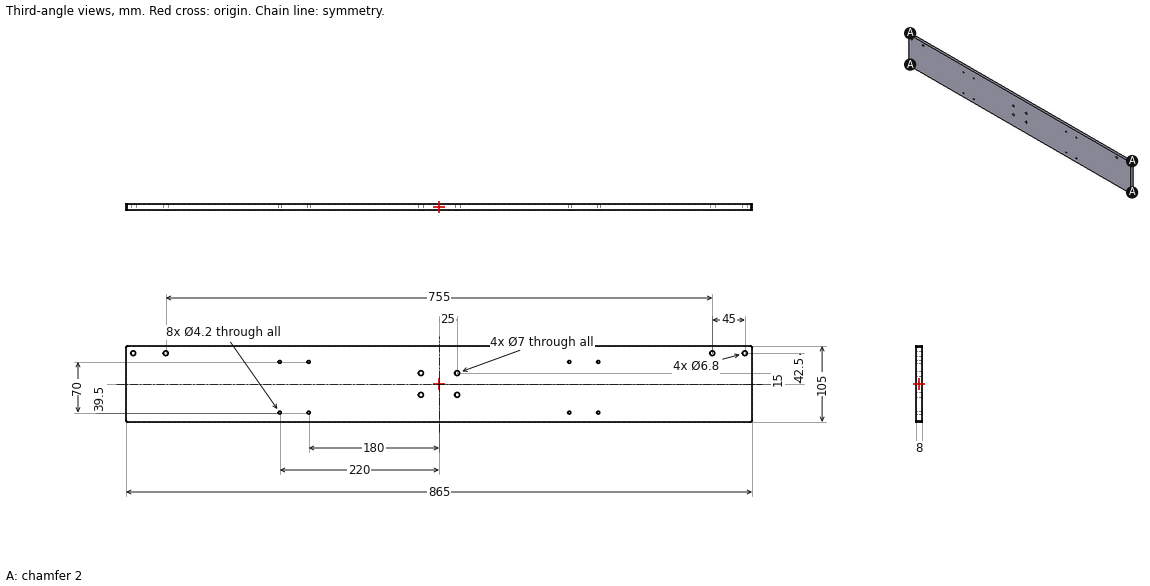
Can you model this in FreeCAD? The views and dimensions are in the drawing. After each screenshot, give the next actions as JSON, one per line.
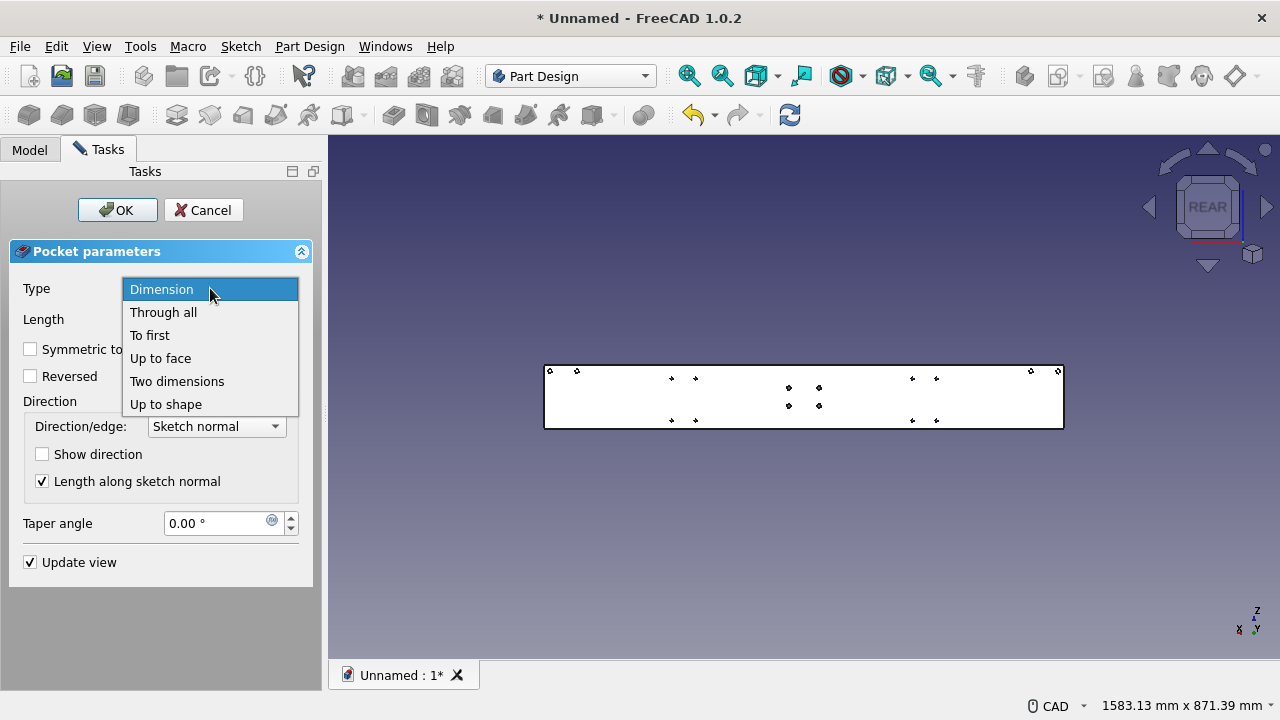
{"action": "left_click", "coordinate": [208, 312]}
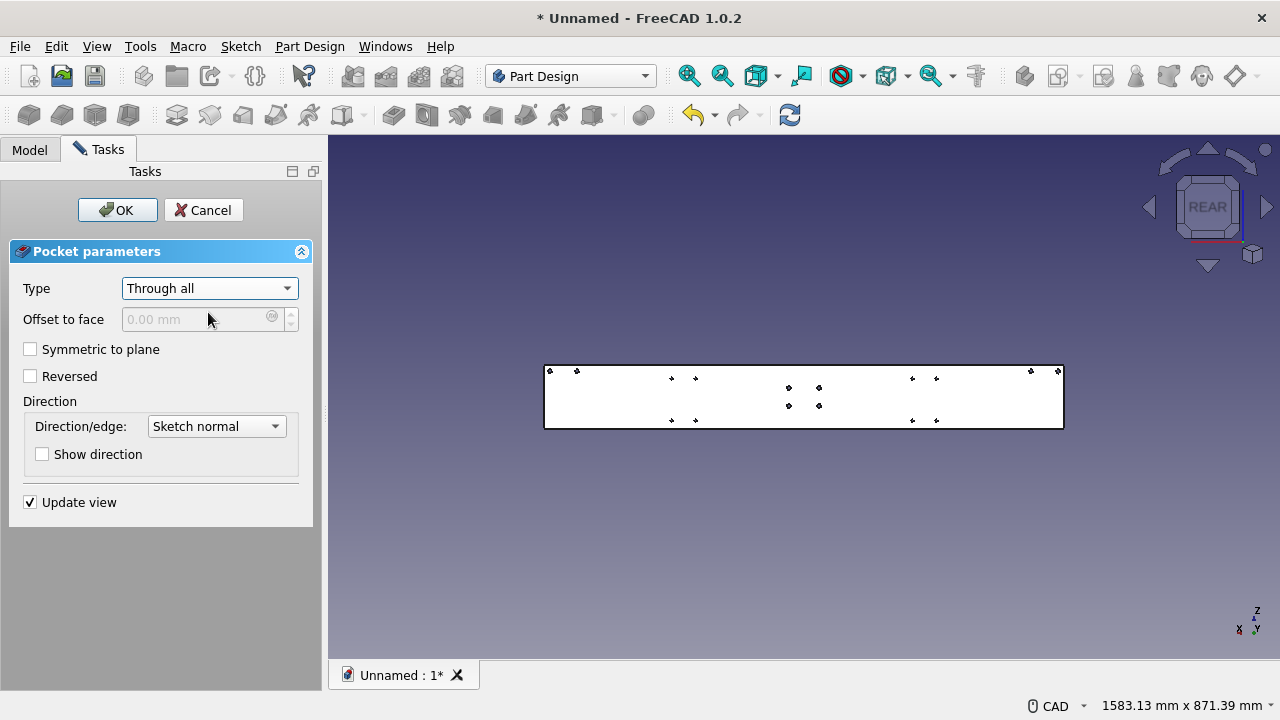
{"action": "left_click", "coordinate": [118, 210]}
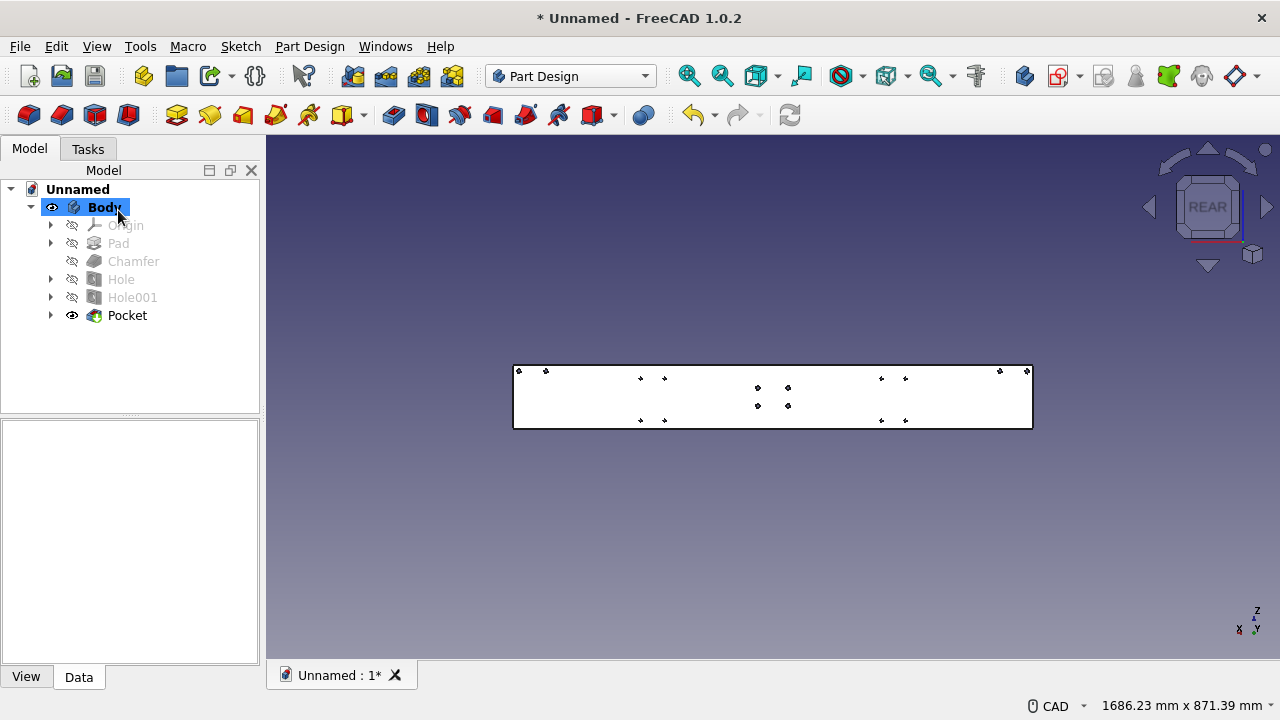
{"action": "key", "text": "0"}